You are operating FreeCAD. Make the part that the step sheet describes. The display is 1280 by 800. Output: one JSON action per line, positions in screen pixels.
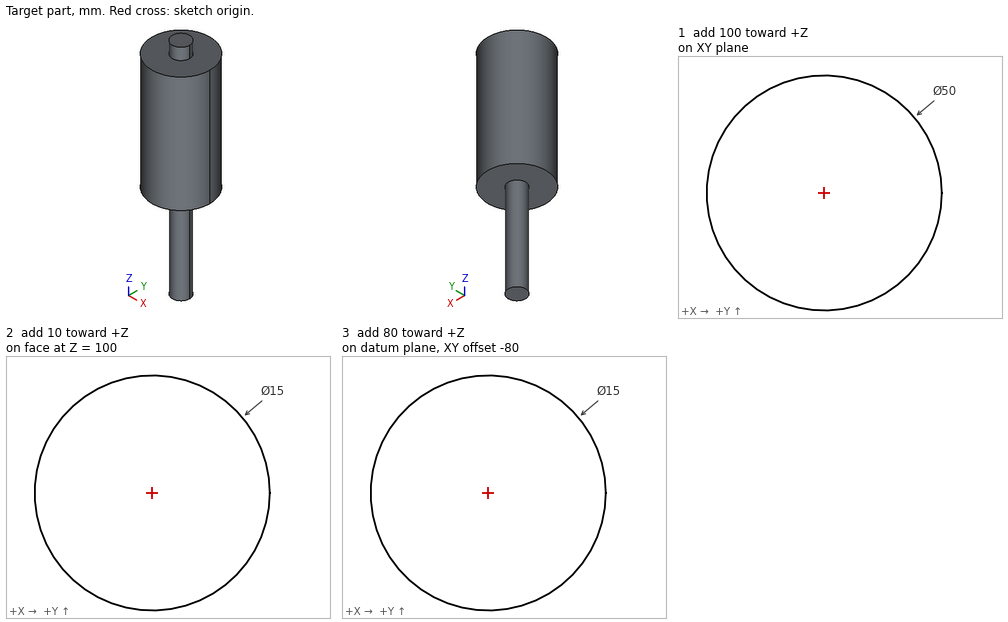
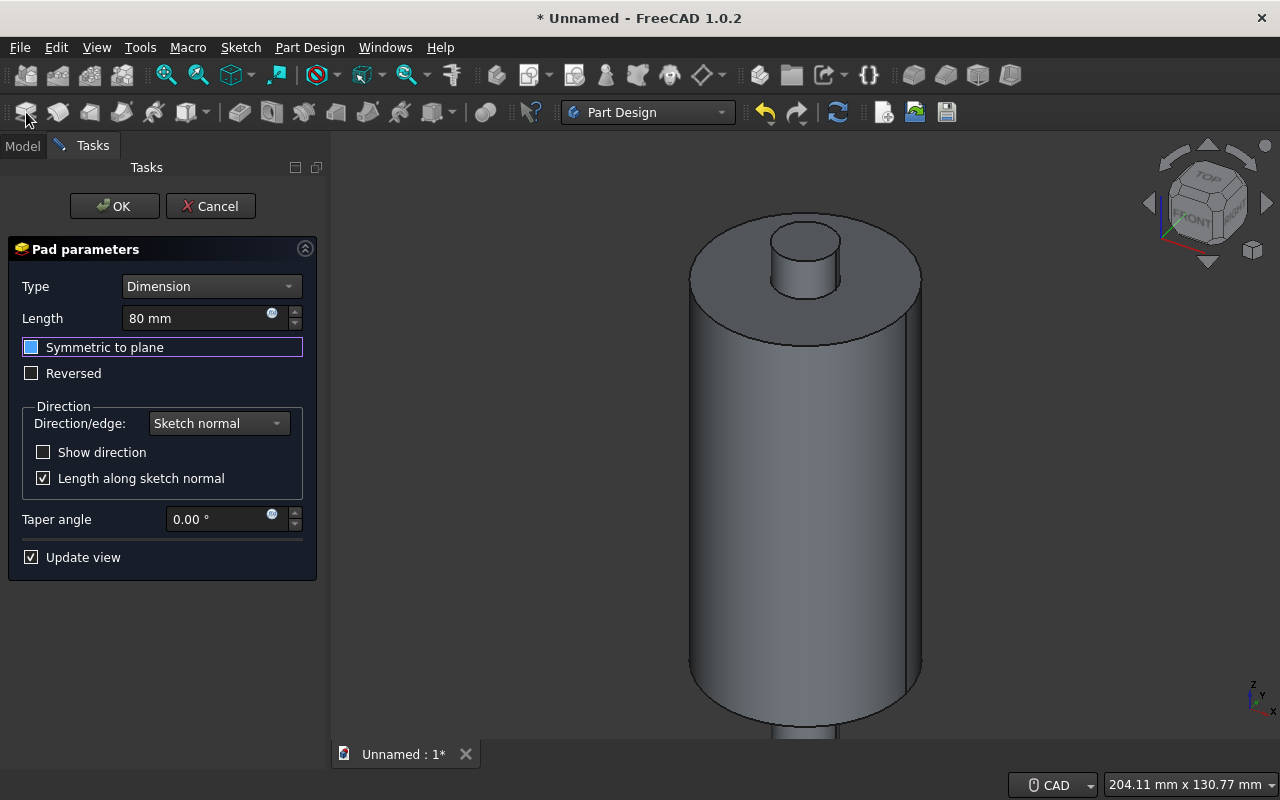
{"action": "left_click", "coordinate": [115, 206]}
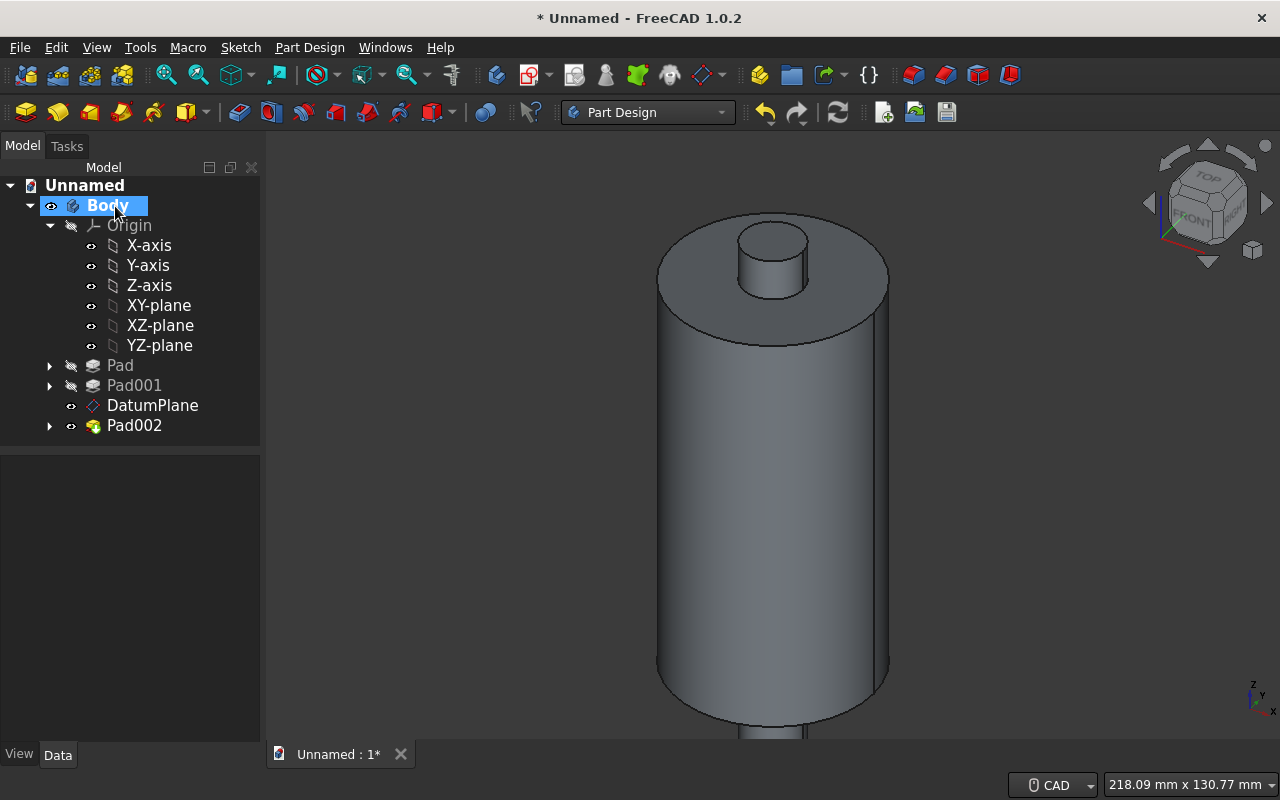
{"action": "left_click", "coordinate": [116, 406]}
{"action": "key", "text": "space"}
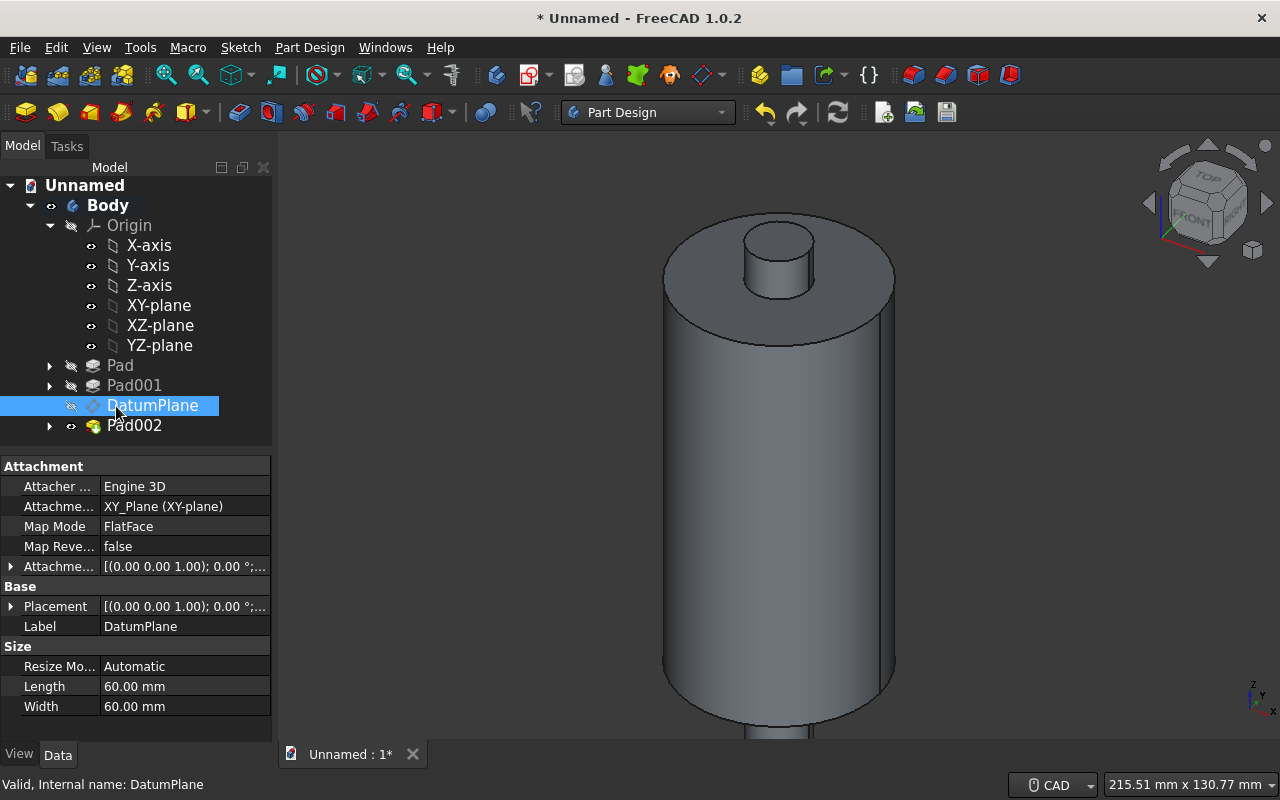
{"action": "key", "text": "0"}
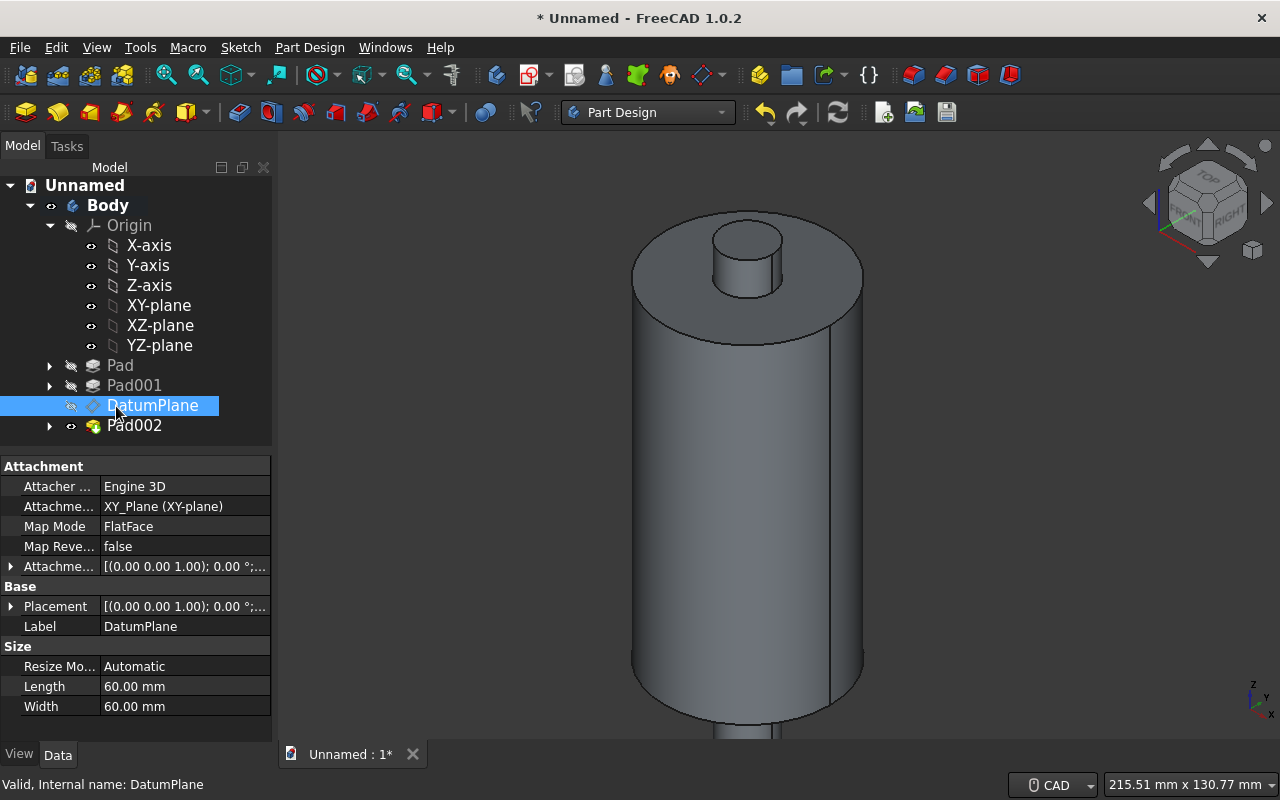
{"action": "left_click", "coordinate": [168, 76]}